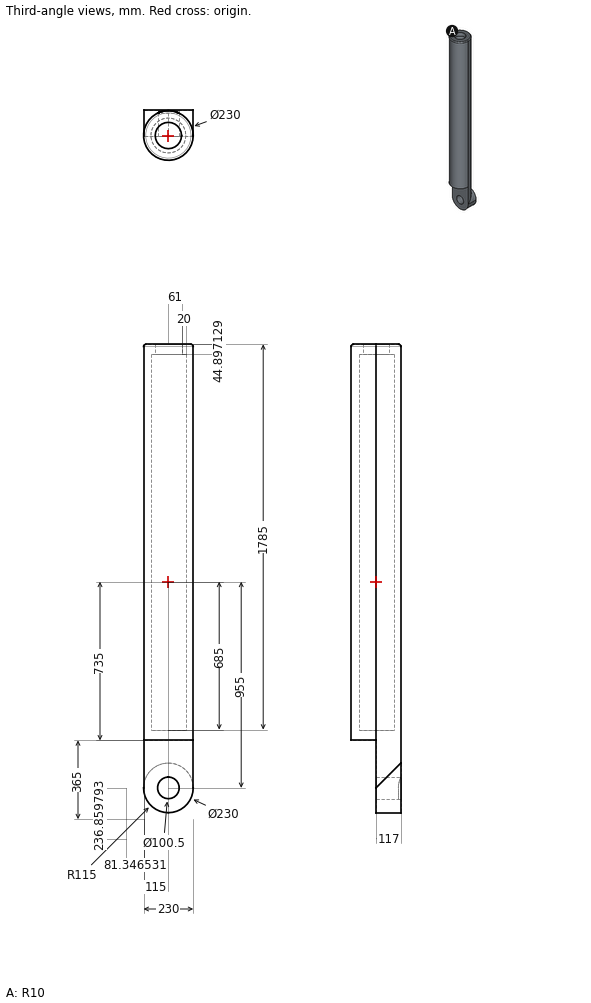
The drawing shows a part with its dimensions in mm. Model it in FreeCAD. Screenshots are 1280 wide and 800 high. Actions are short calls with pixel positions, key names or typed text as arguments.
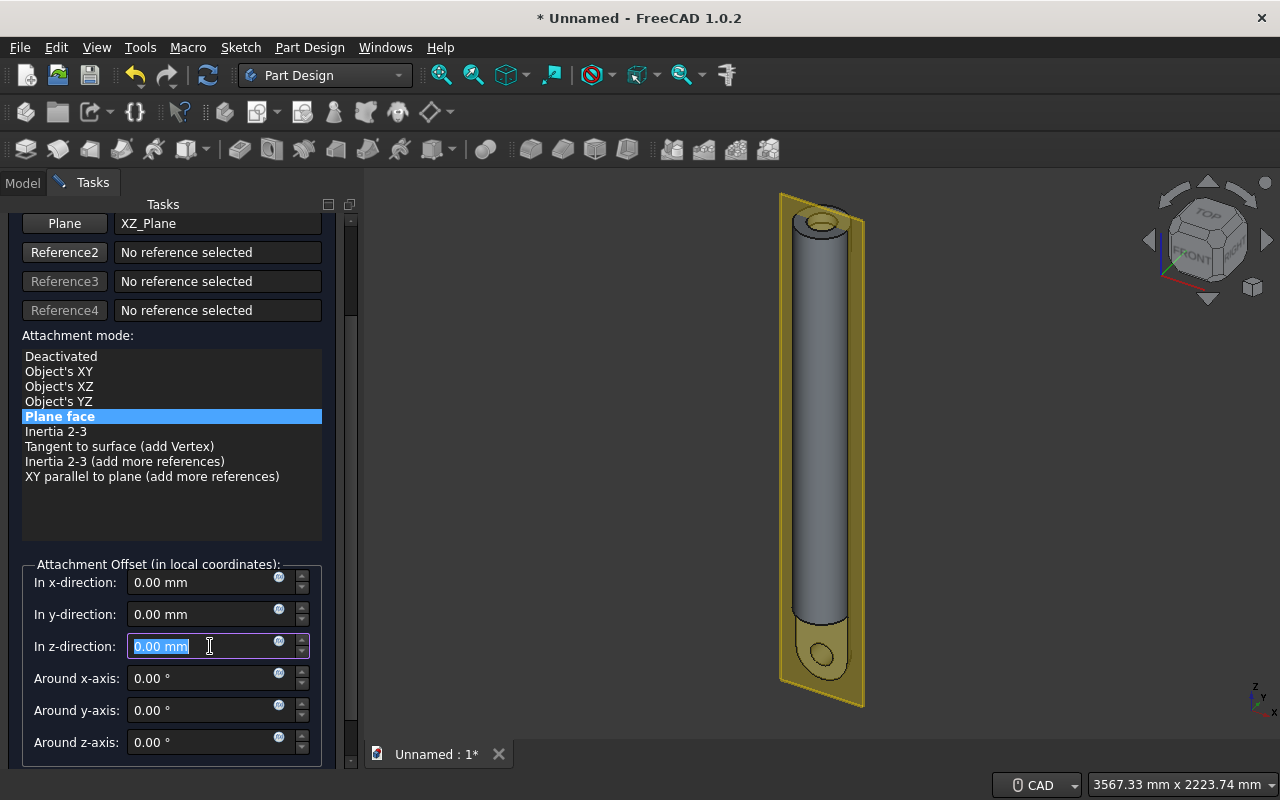
text(-117)
key(Tab)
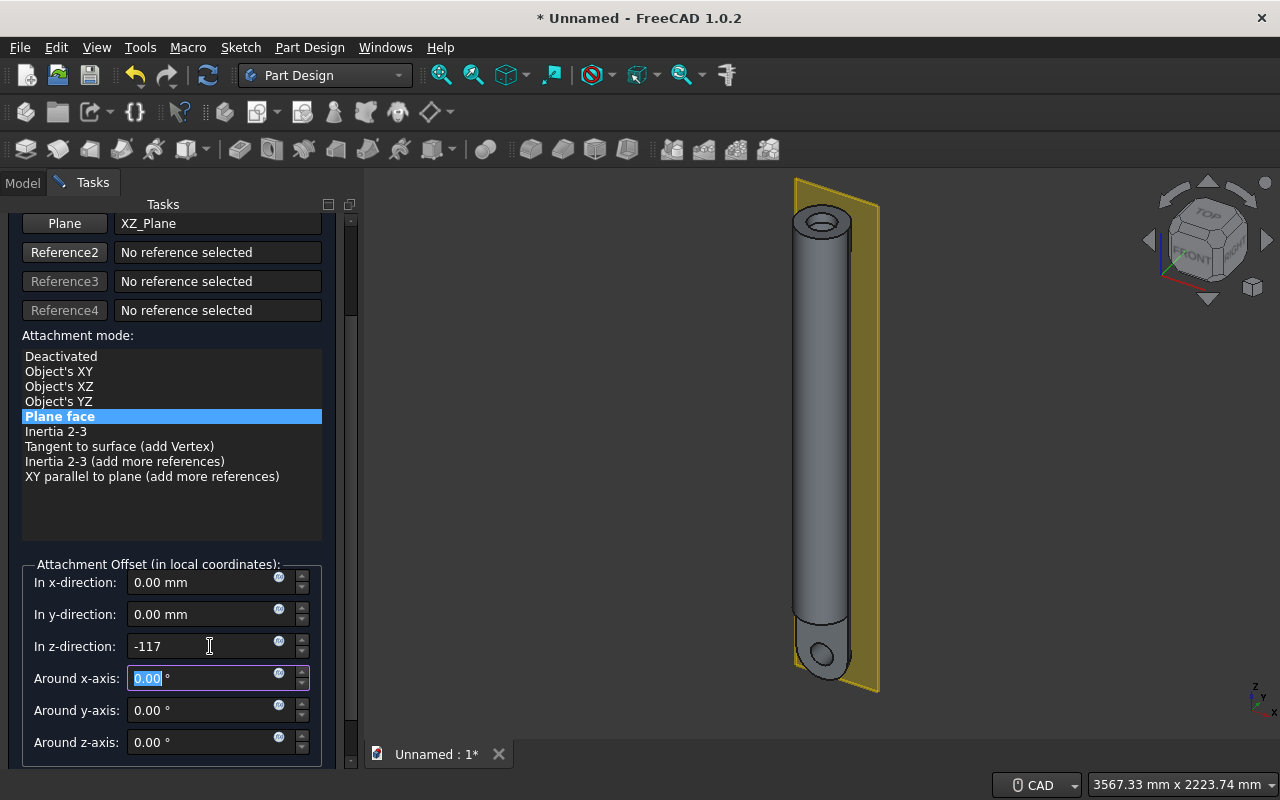
scroll(351, 491, up, 3)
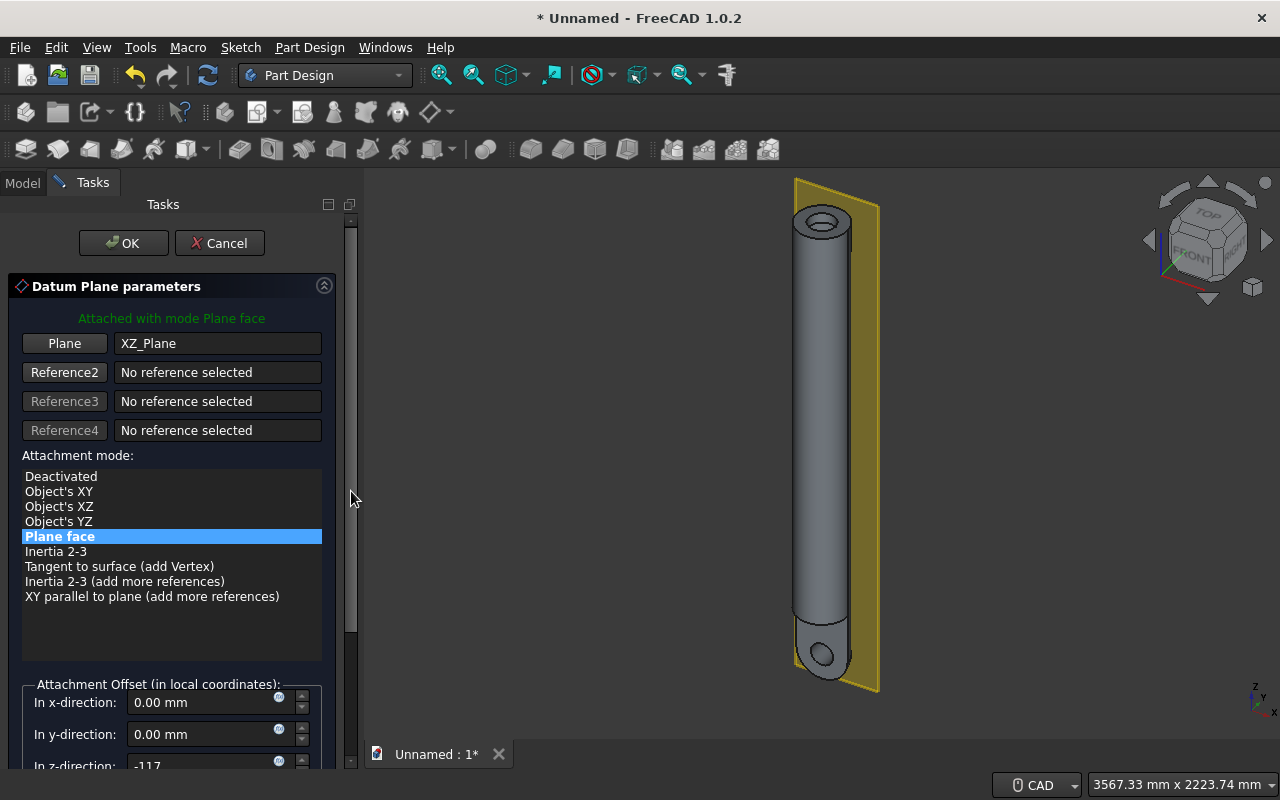
click(124, 243)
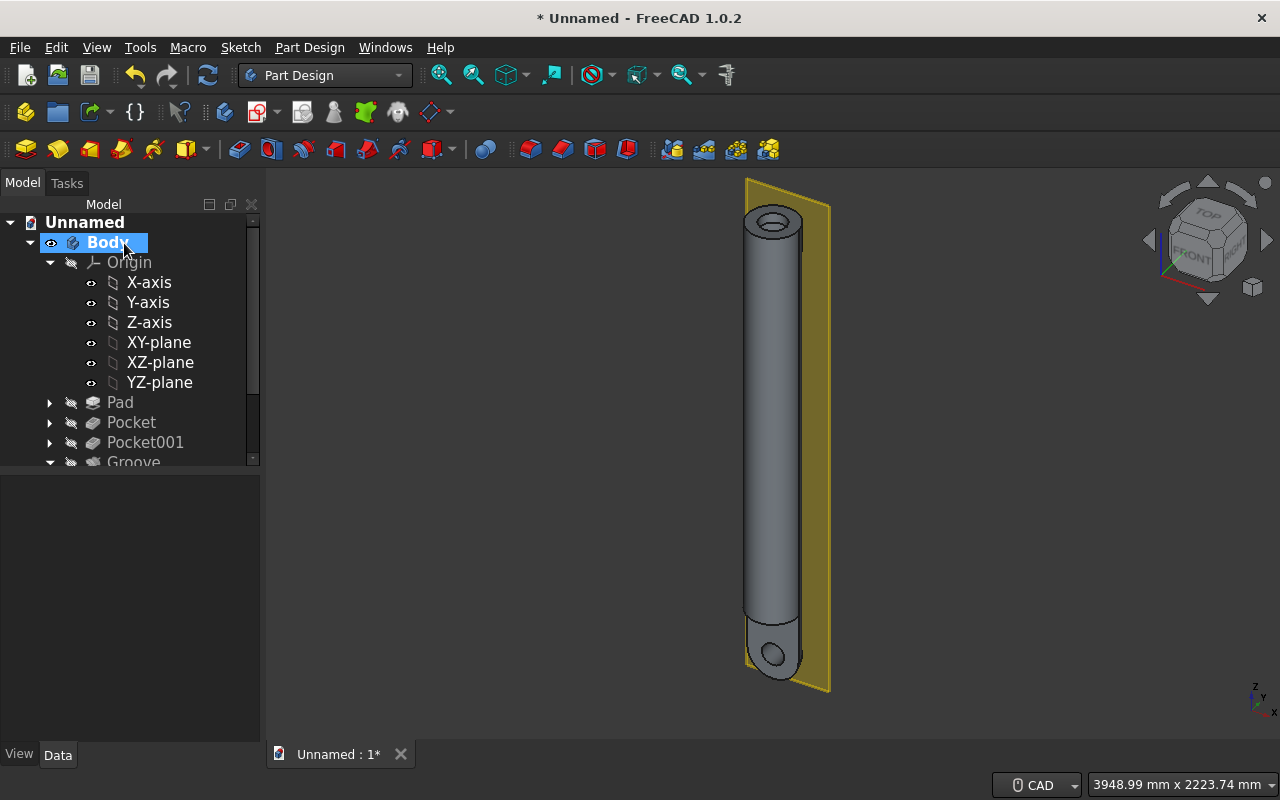
scroll(100, 338, down, 3)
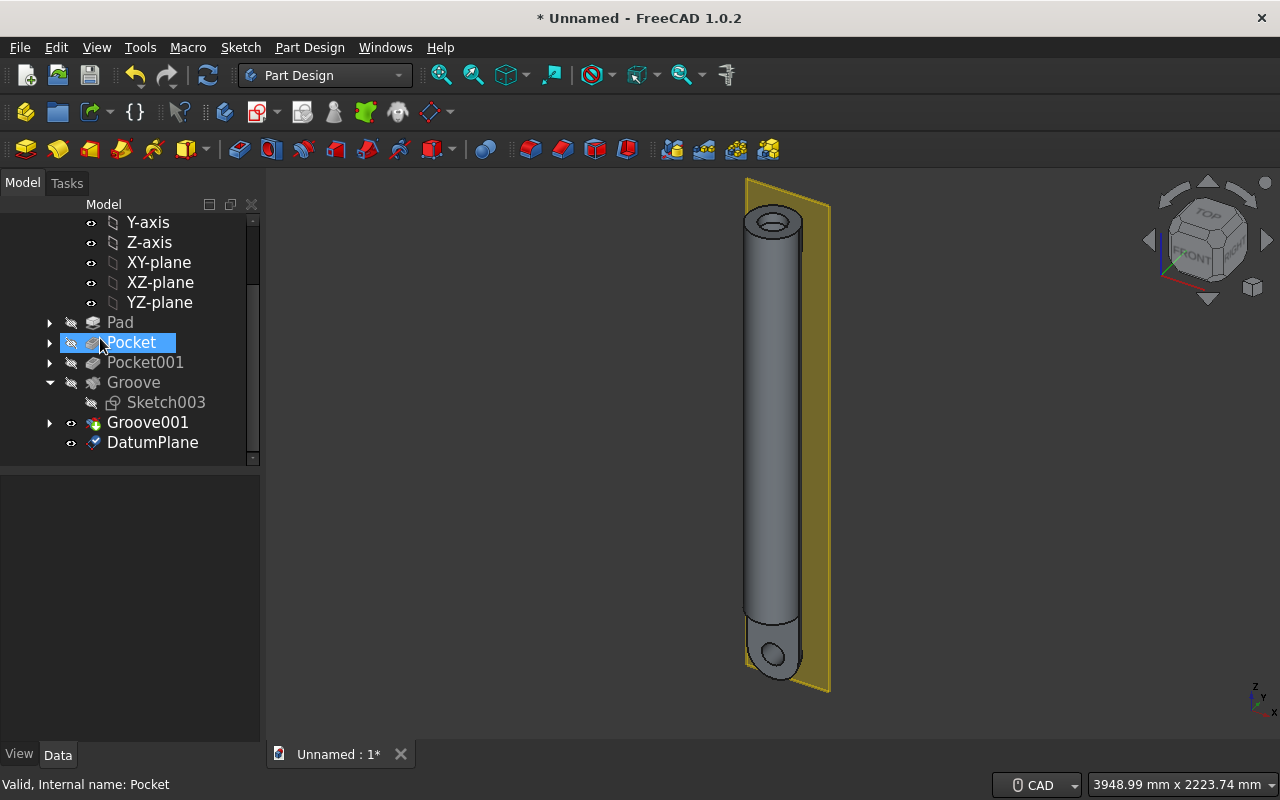
click(116, 443)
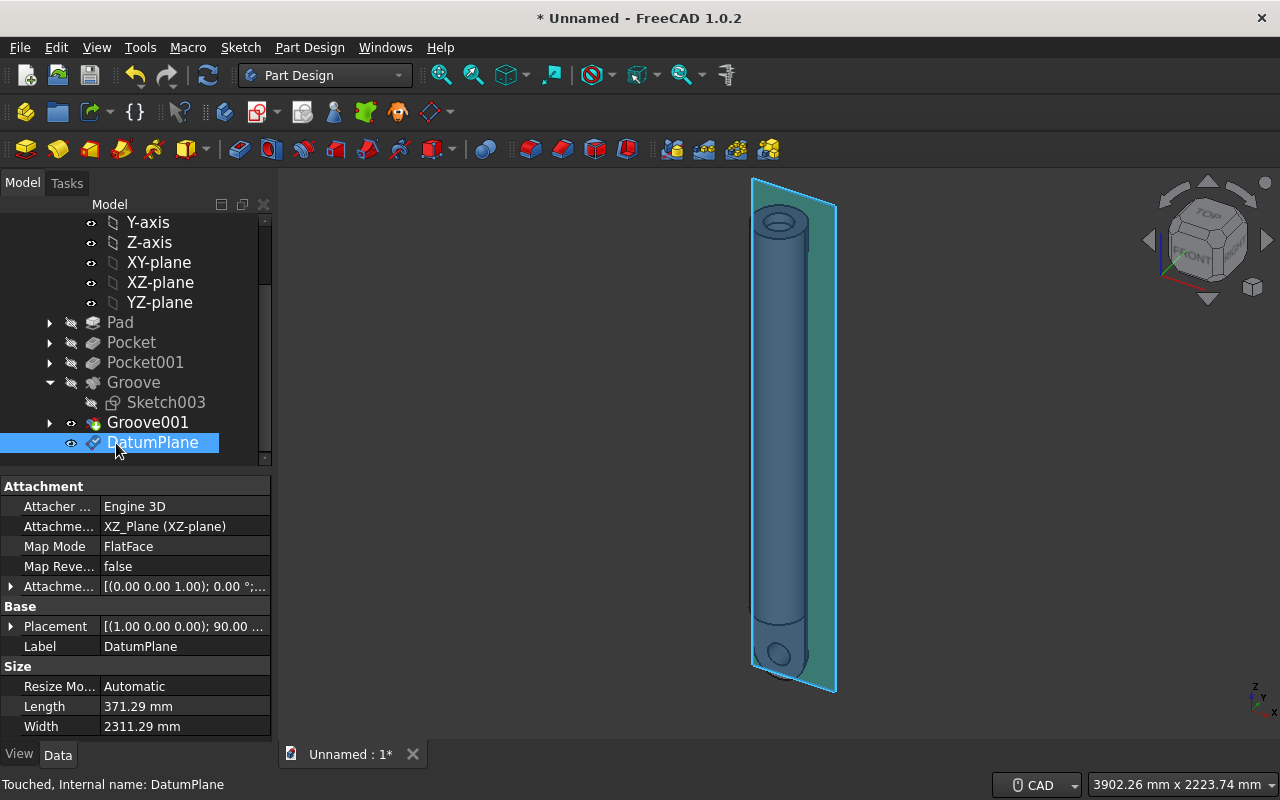
click(258, 112)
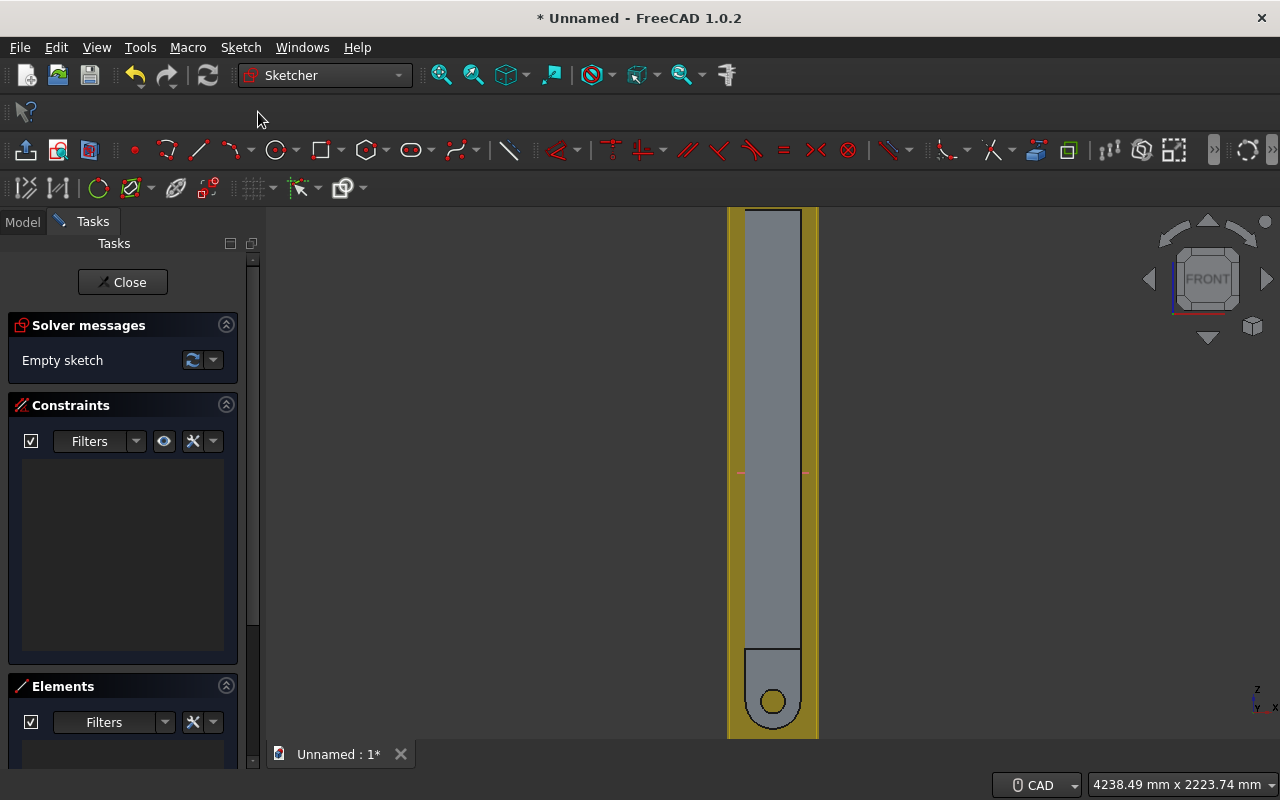
click(90, 150)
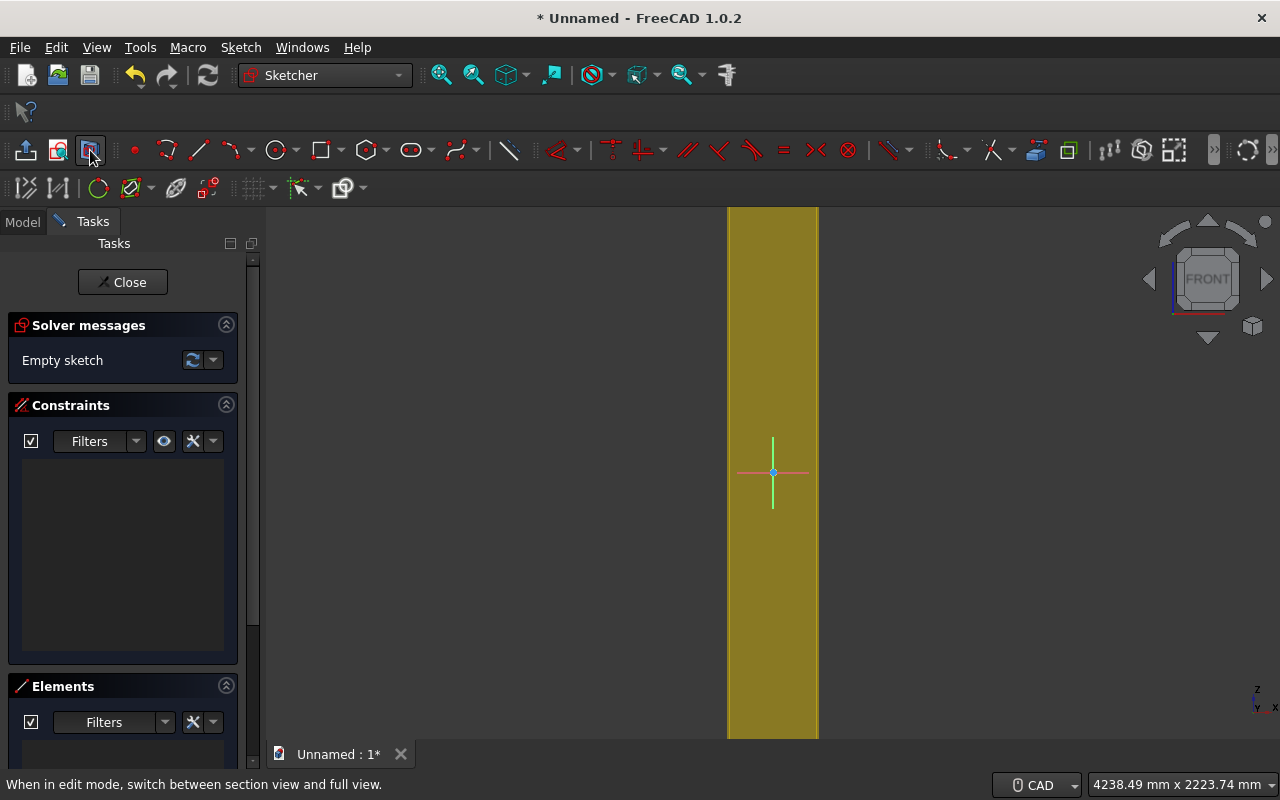
scroll(704, 473, down, 5)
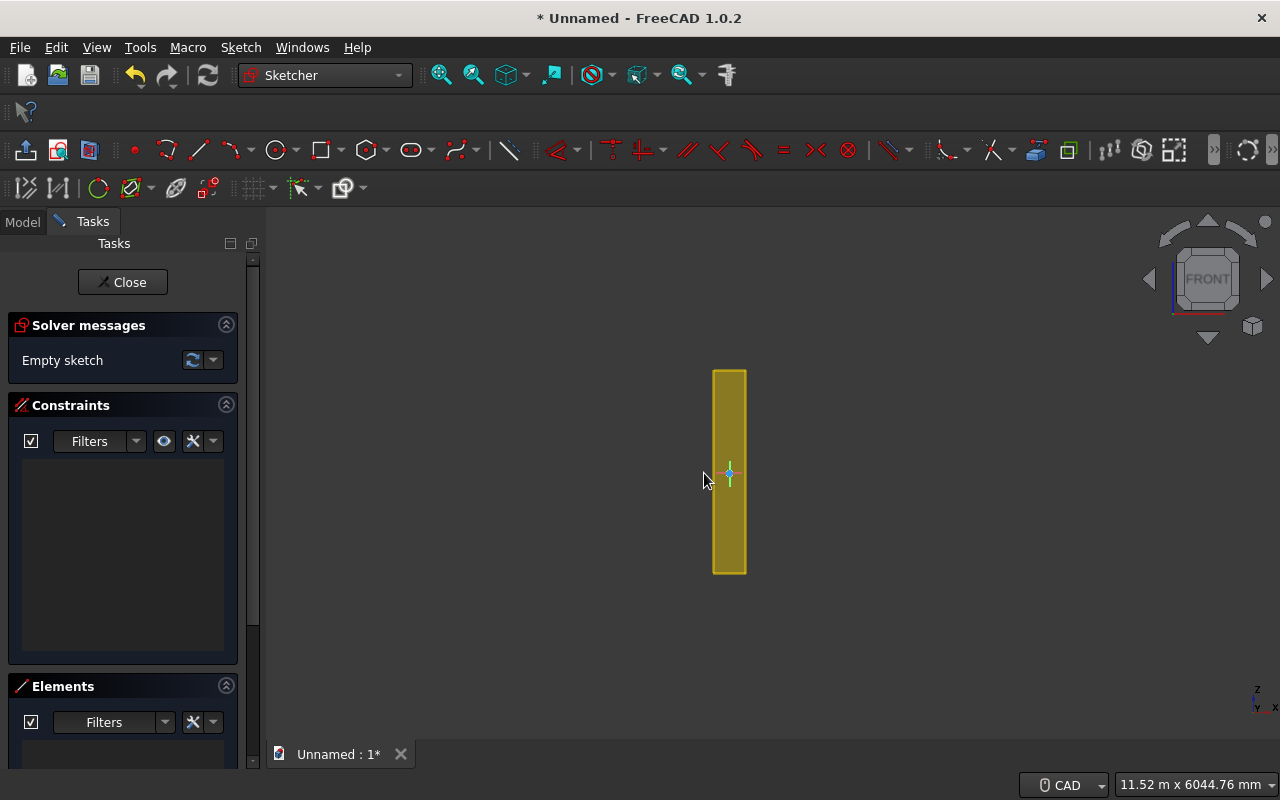
scroll(731, 563, up, 14)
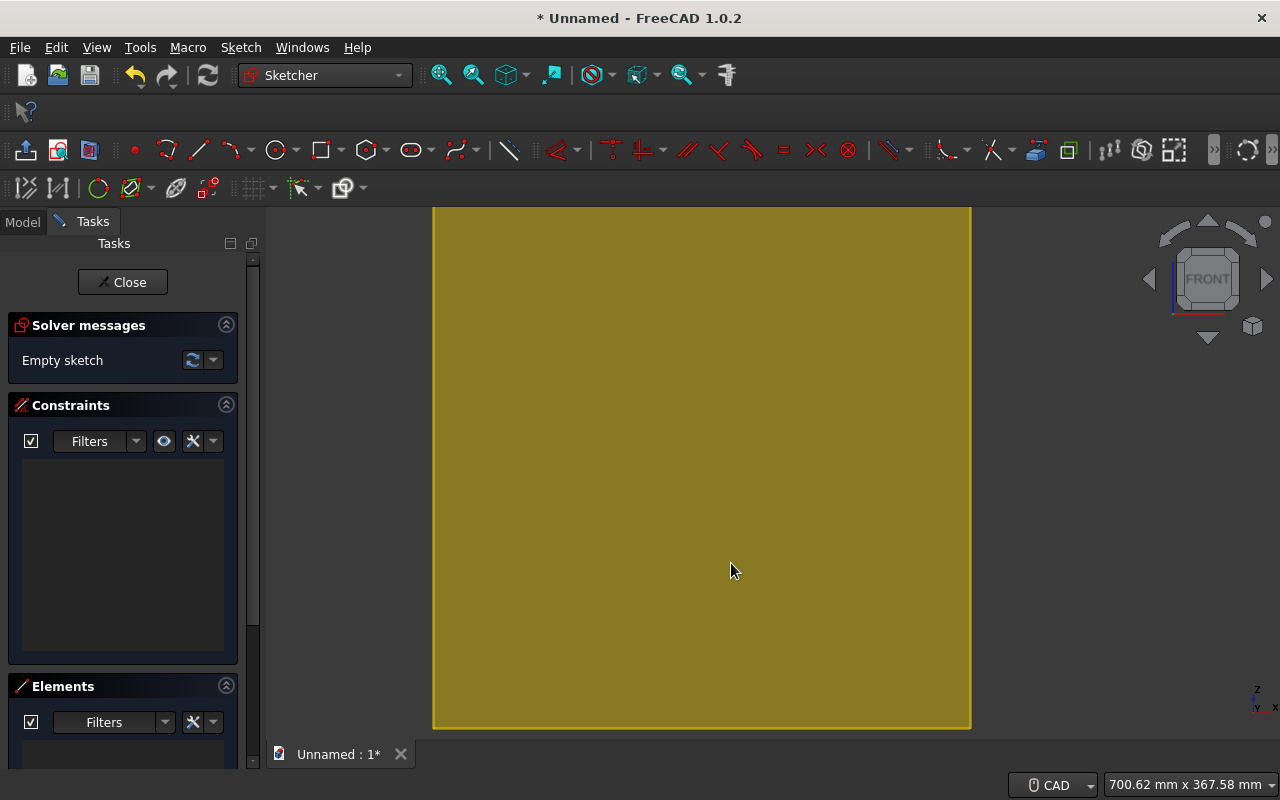
click(276, 150)